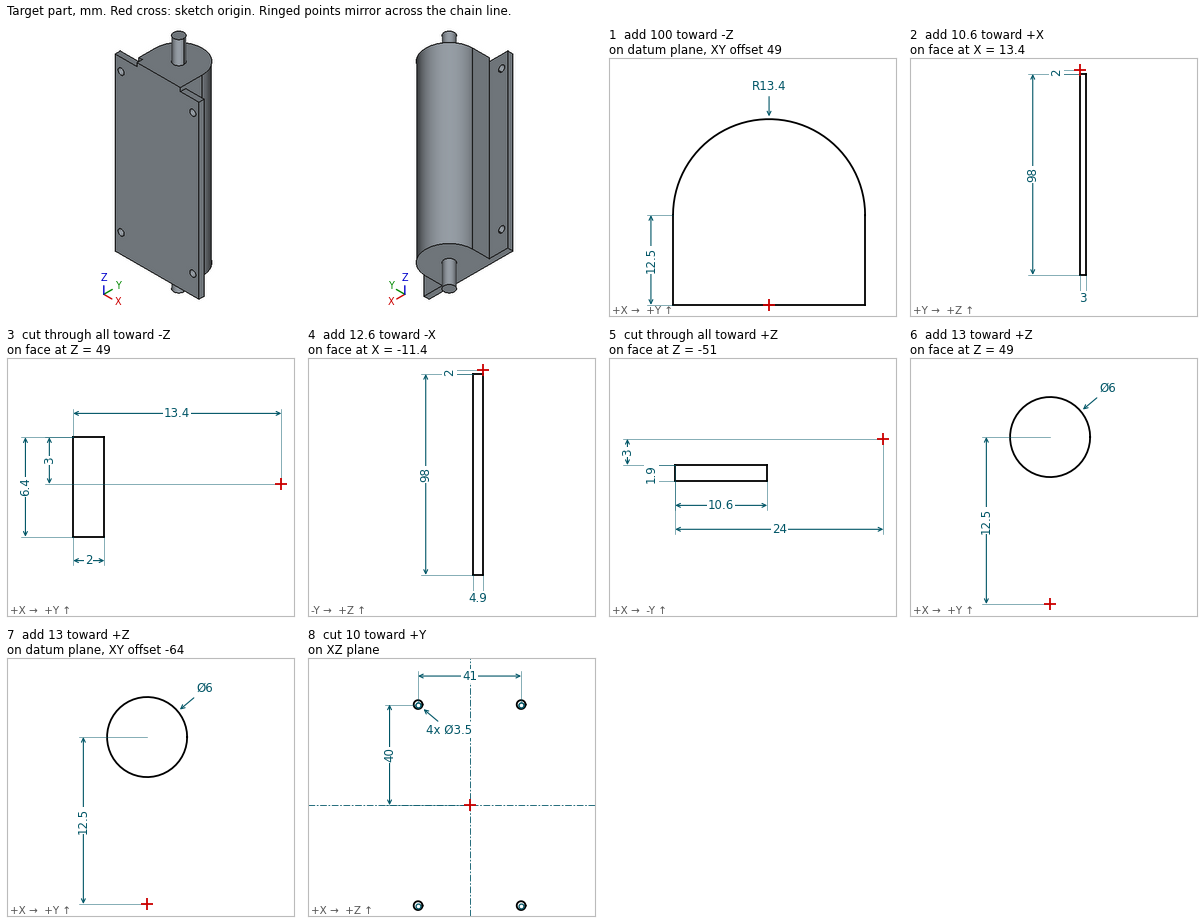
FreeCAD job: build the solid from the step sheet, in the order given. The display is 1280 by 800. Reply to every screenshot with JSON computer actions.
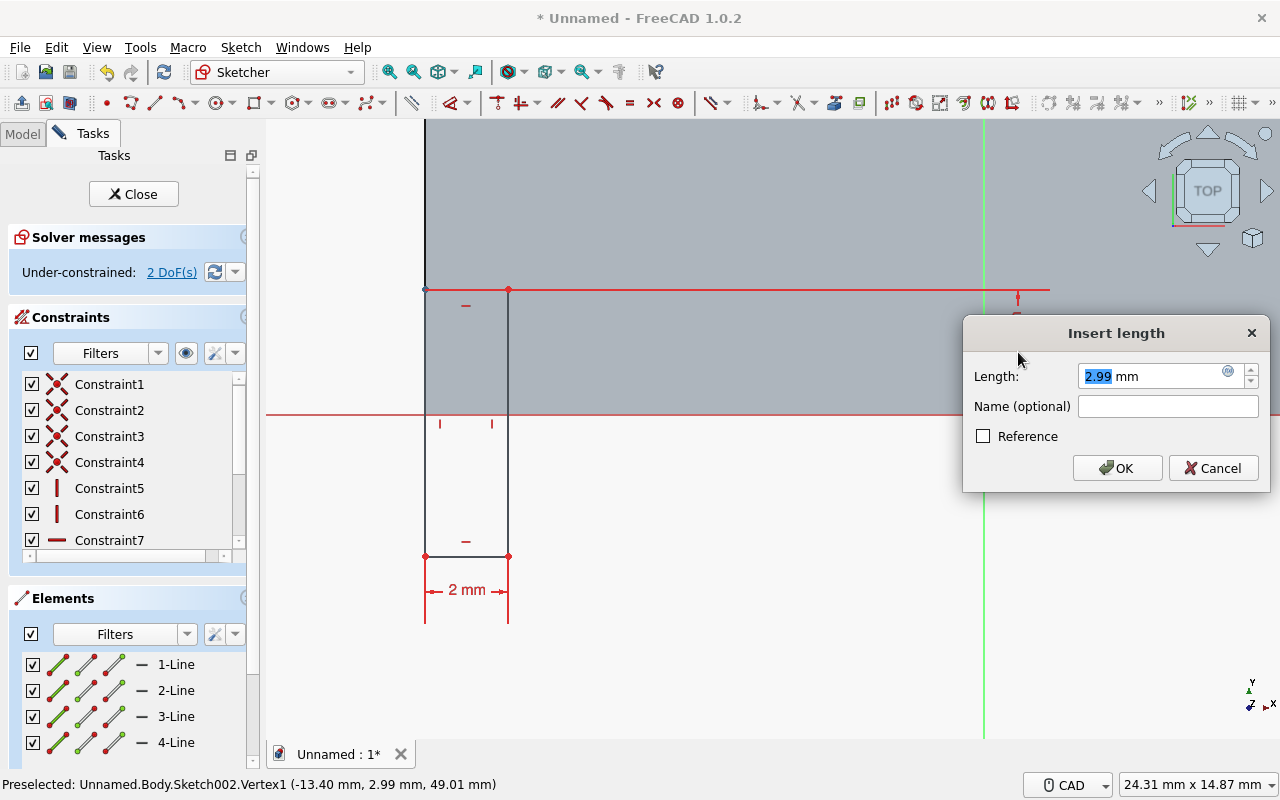
{"action": "type", "text": "3"}
{"action": "key", "text": "Return"}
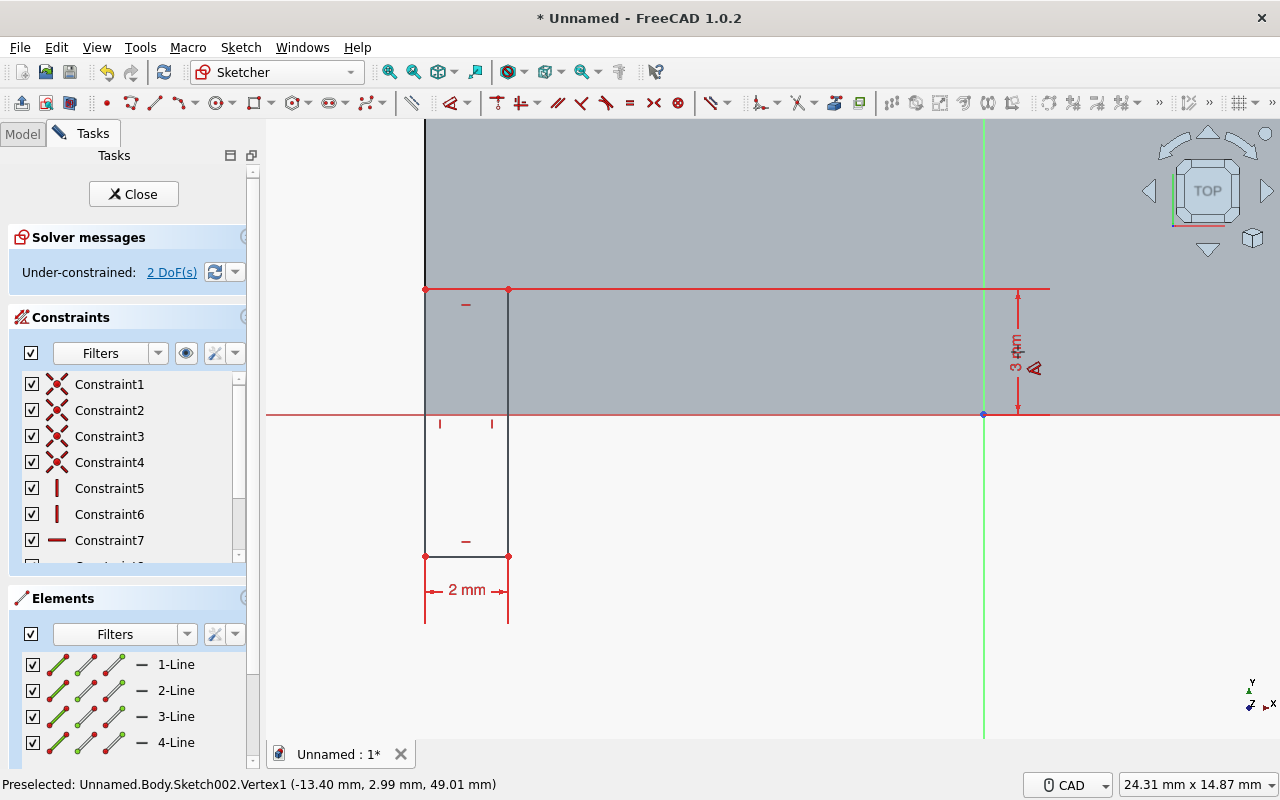
{"action": "left_click", "coordinate": [425, 370]}
{"action": "left_click", "coordinate": [391, 362]}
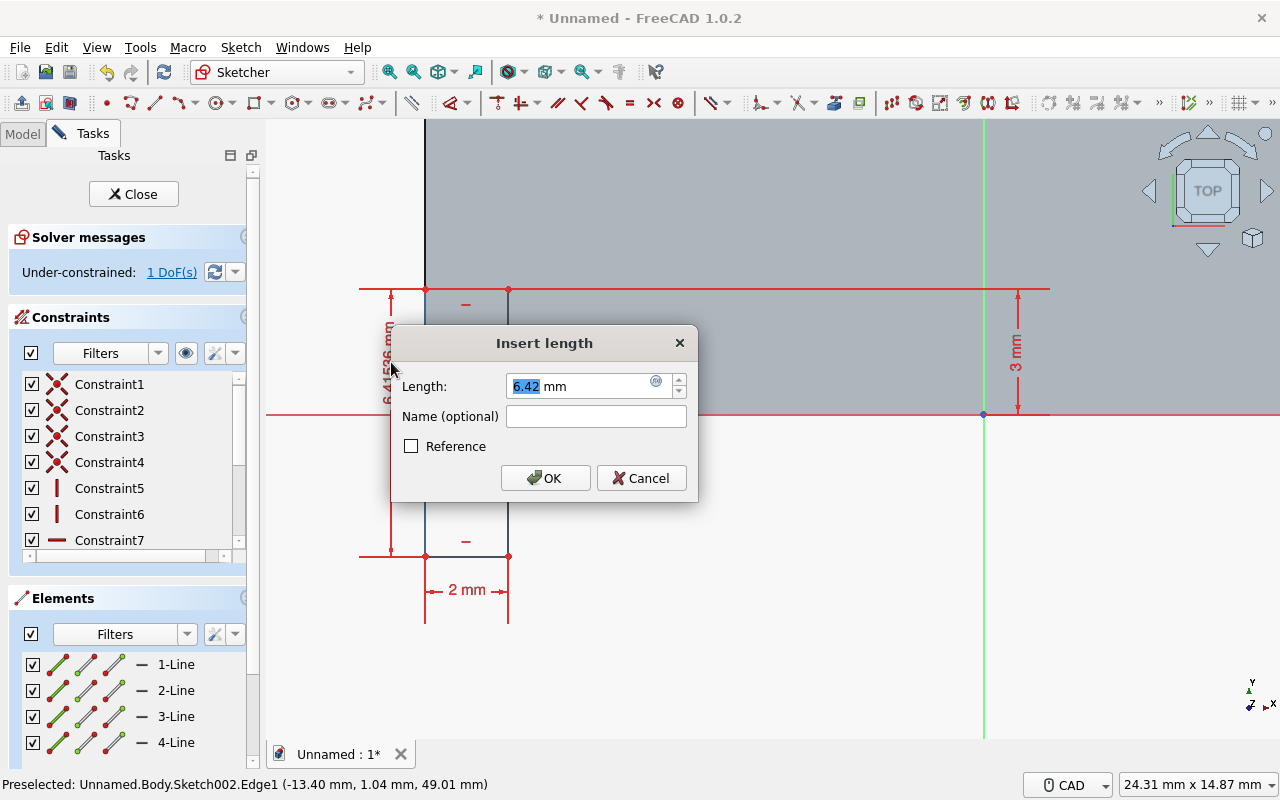
{"action": "type", "text": "6.4"}
{"action": "key", "text": "Return"}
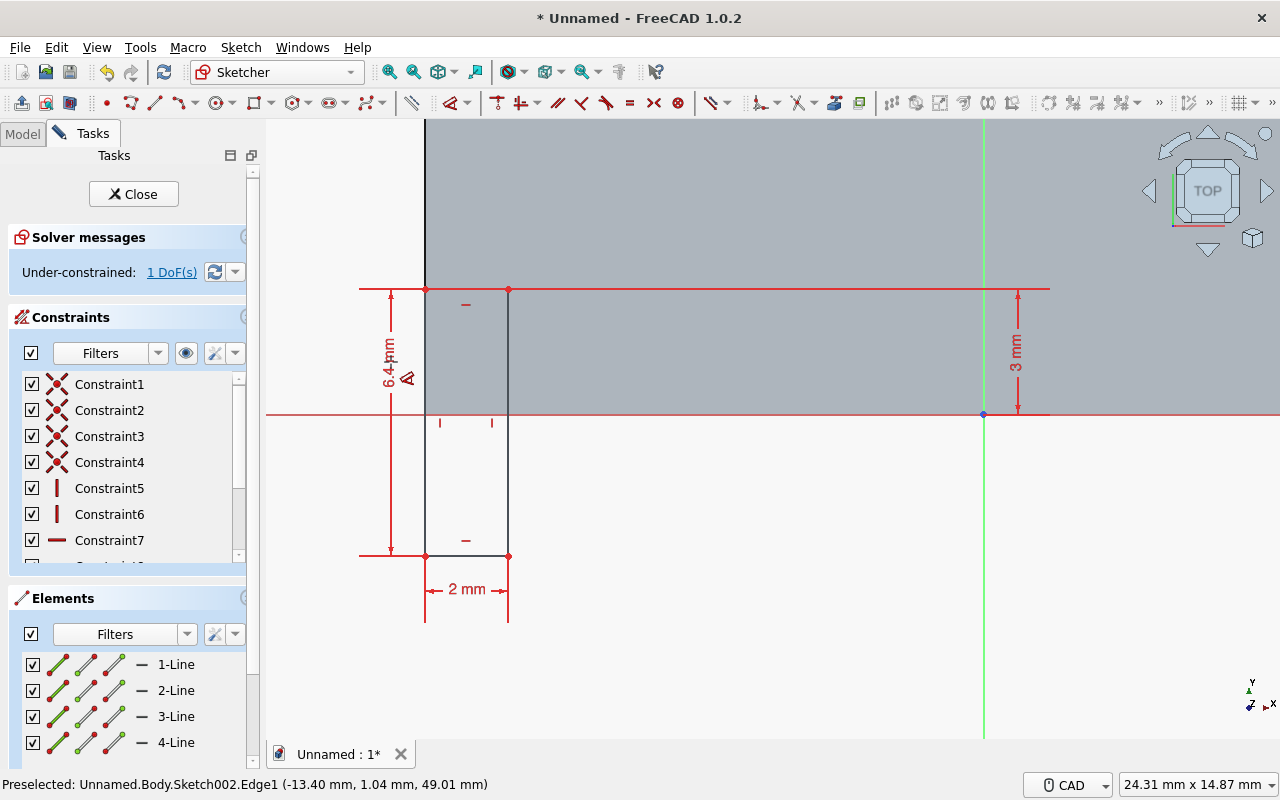
{"action": "left_click", "coordinate": [425, 289]}
{"action": "left_click", "coordinate": [704, 255]}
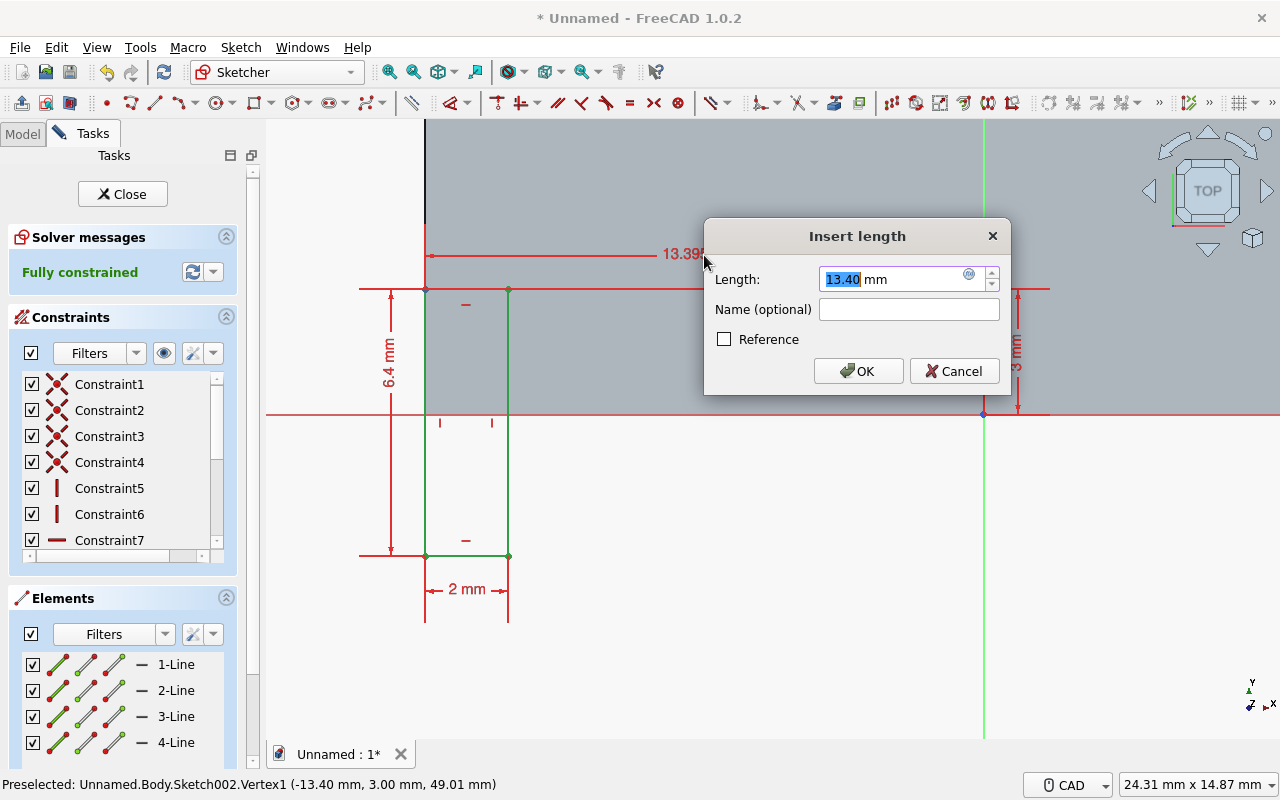
{"action": "type", "text": "13.4"}
{"action": "key", "text": "Return"}
{"action": "key", "text": "Escape"}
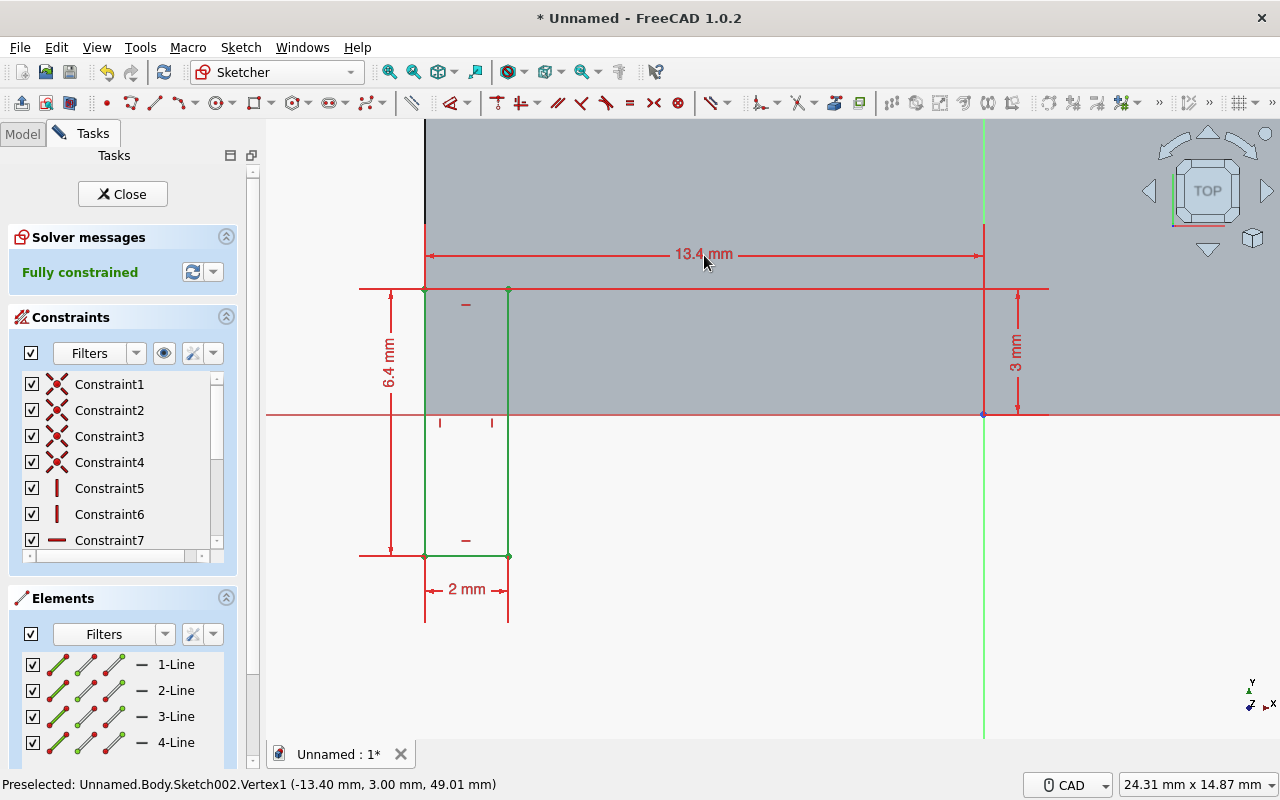
{"action": "left_click", "coordinate": [123, 194]}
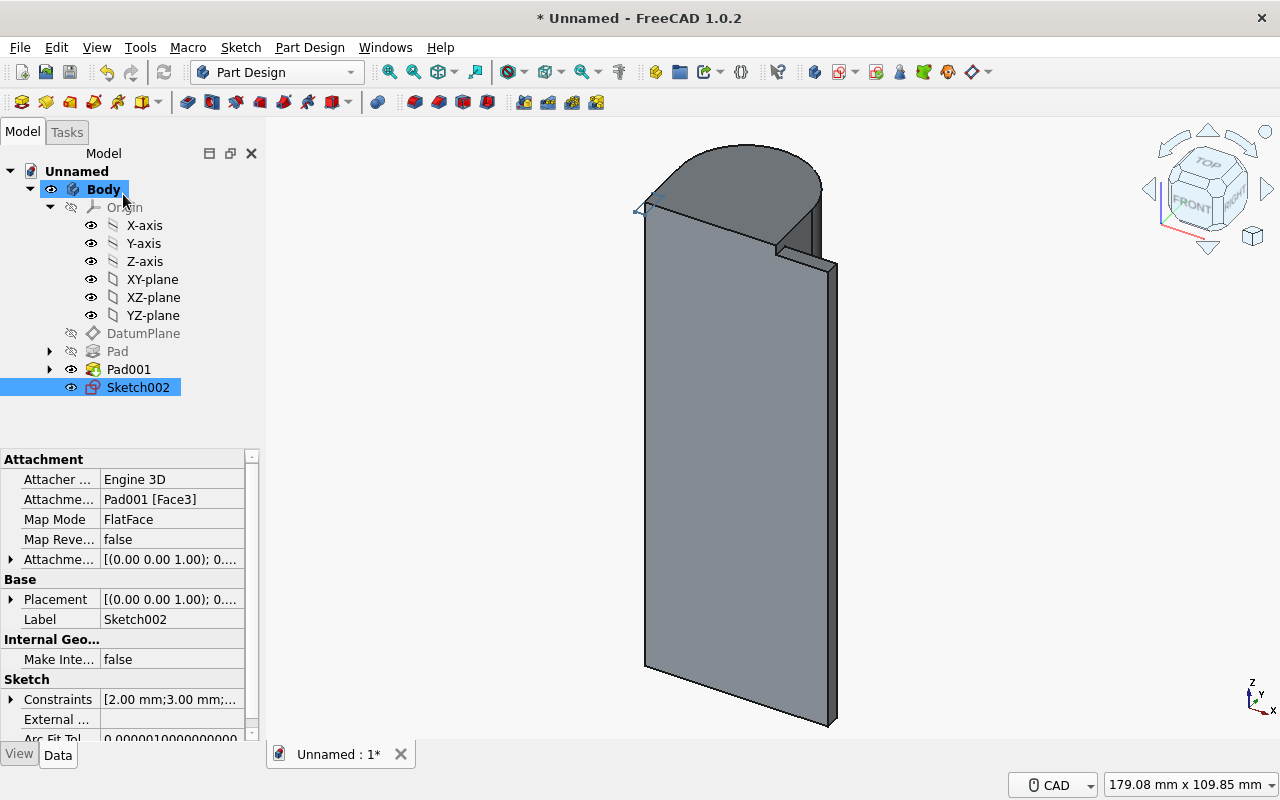
{"action": "left_click", "coordinate": [188, 102]}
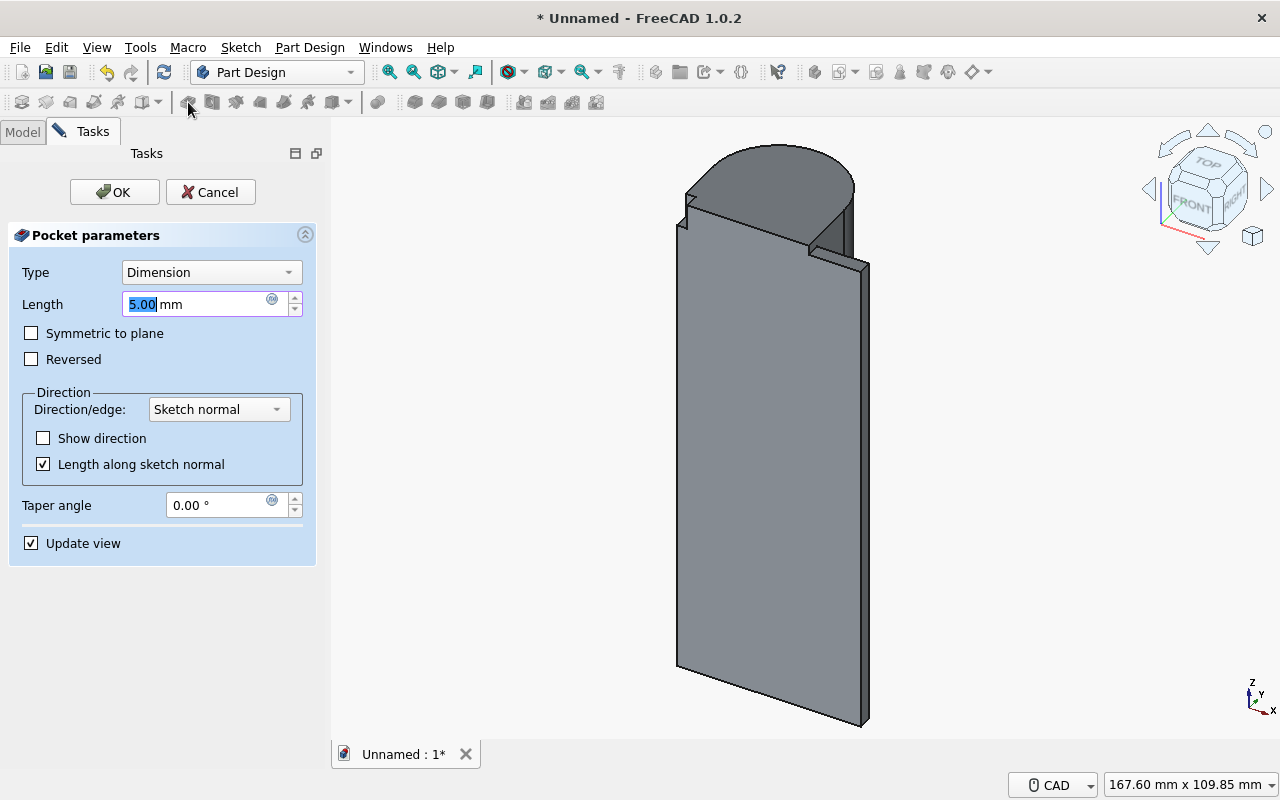
{"action": "left_click", "coordinate": [212, 272]}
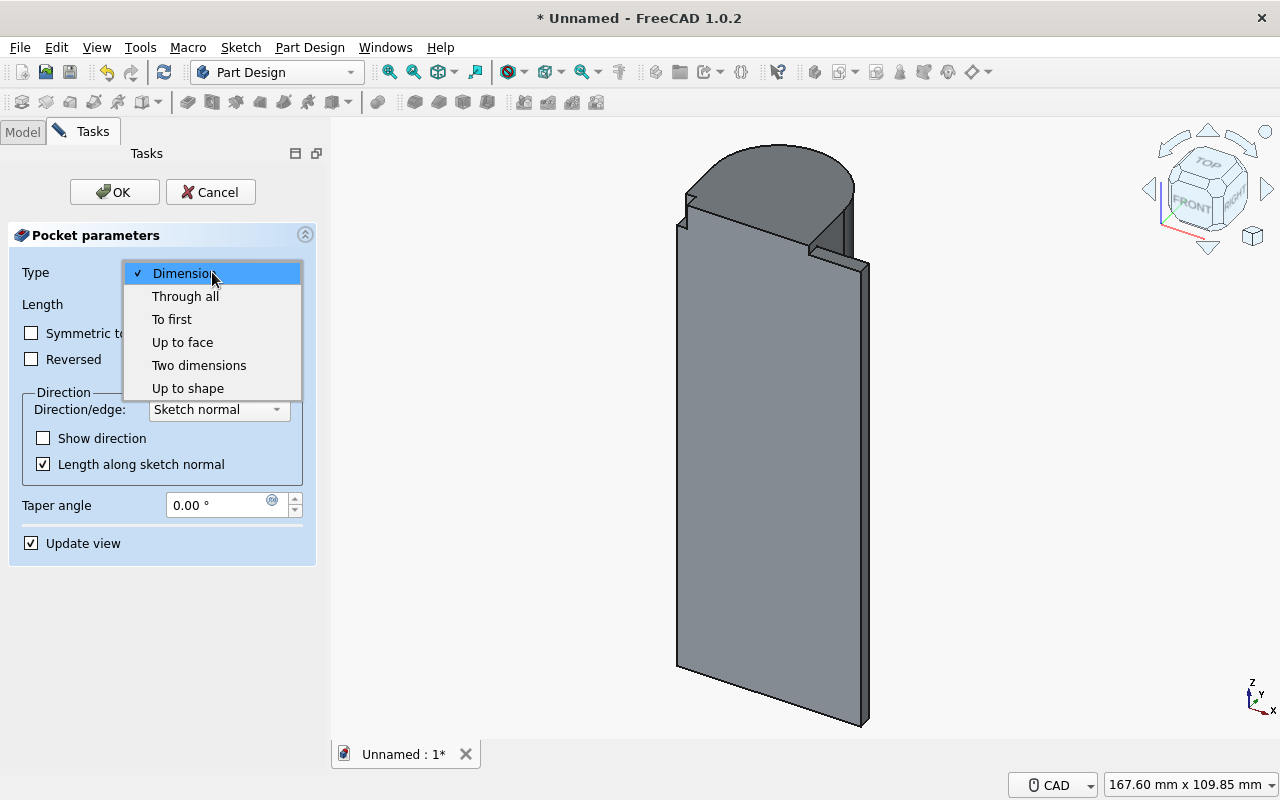
{"action": "left_click", "coordinate": [212, 296]}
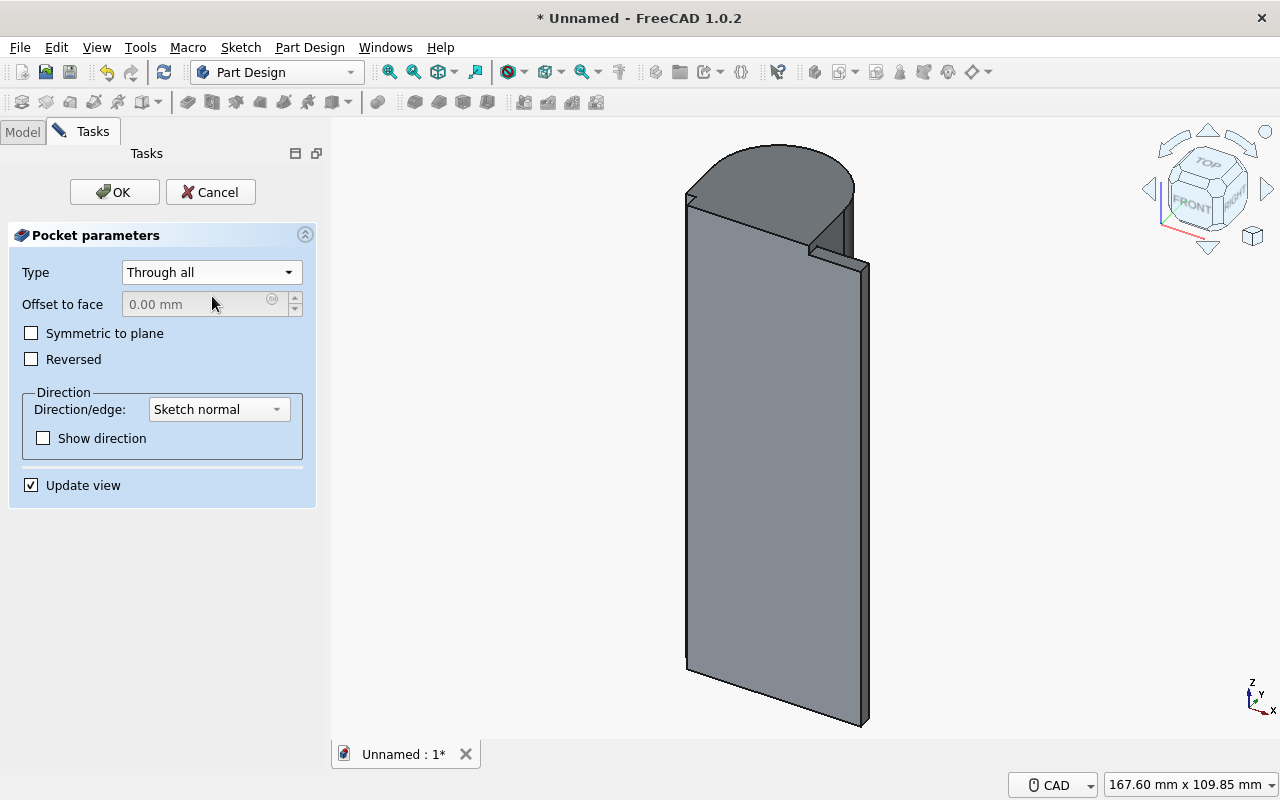
{"action": "left_click", "coordinate": [115, 192]}